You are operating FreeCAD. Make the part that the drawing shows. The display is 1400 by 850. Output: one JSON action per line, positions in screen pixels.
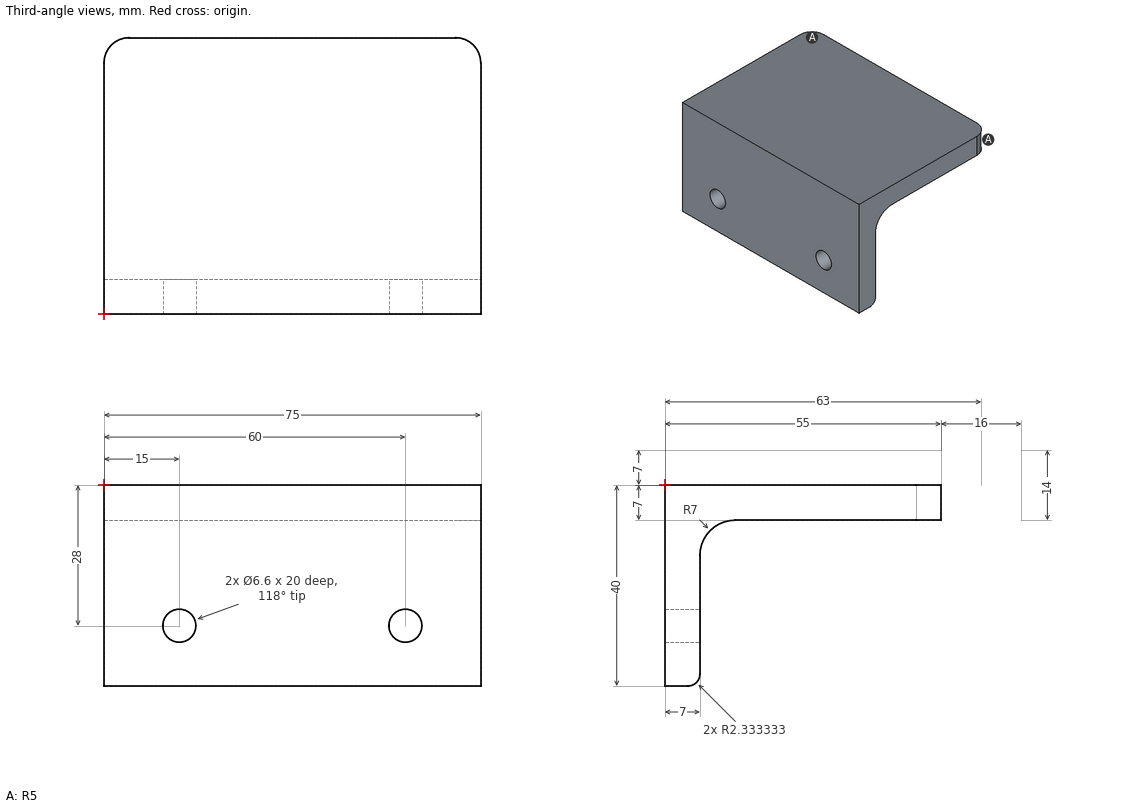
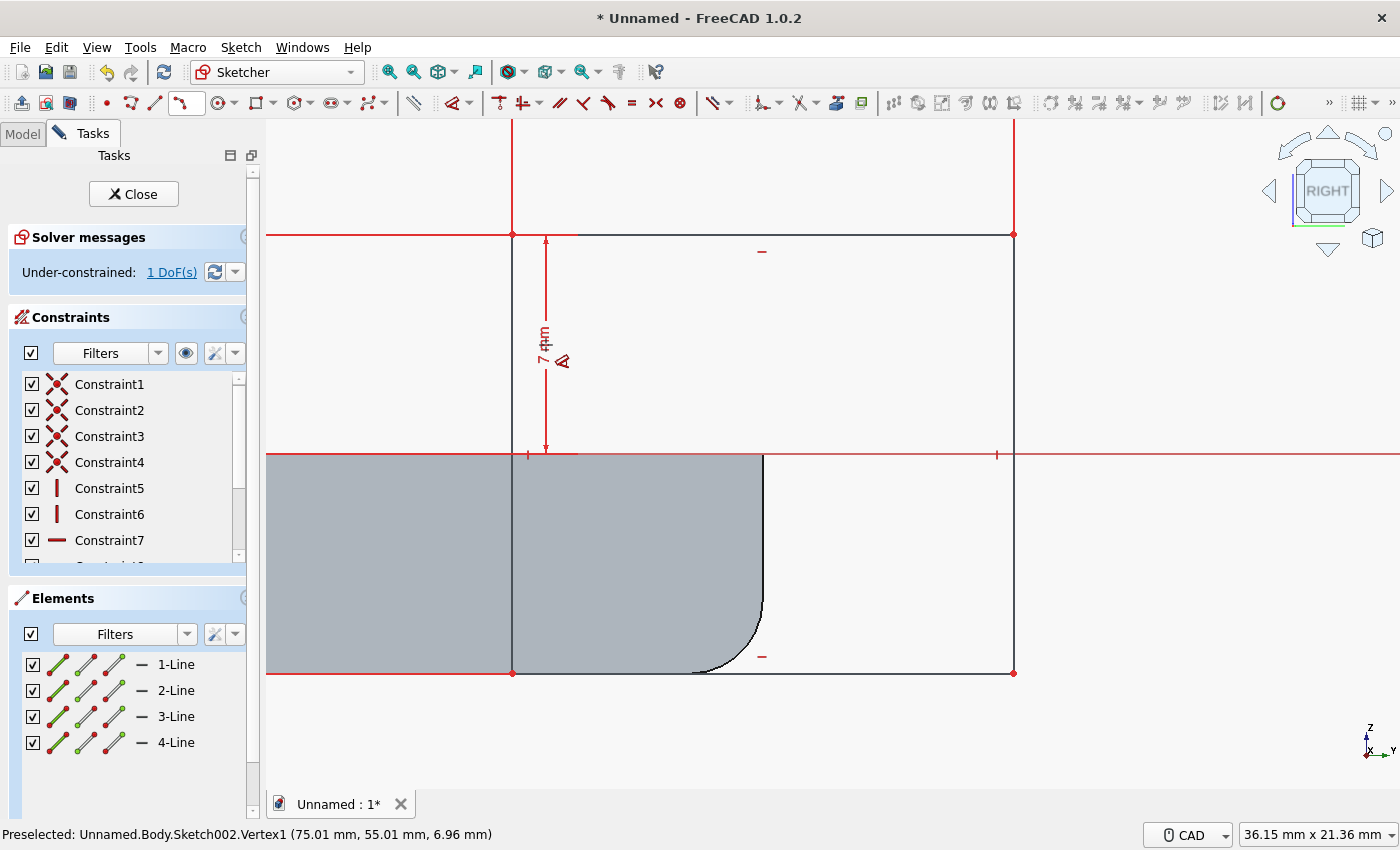
{"action": "left_click", "coordinate": [512, 235]}
{"action": "left_click", "coordinate": [403, 201]}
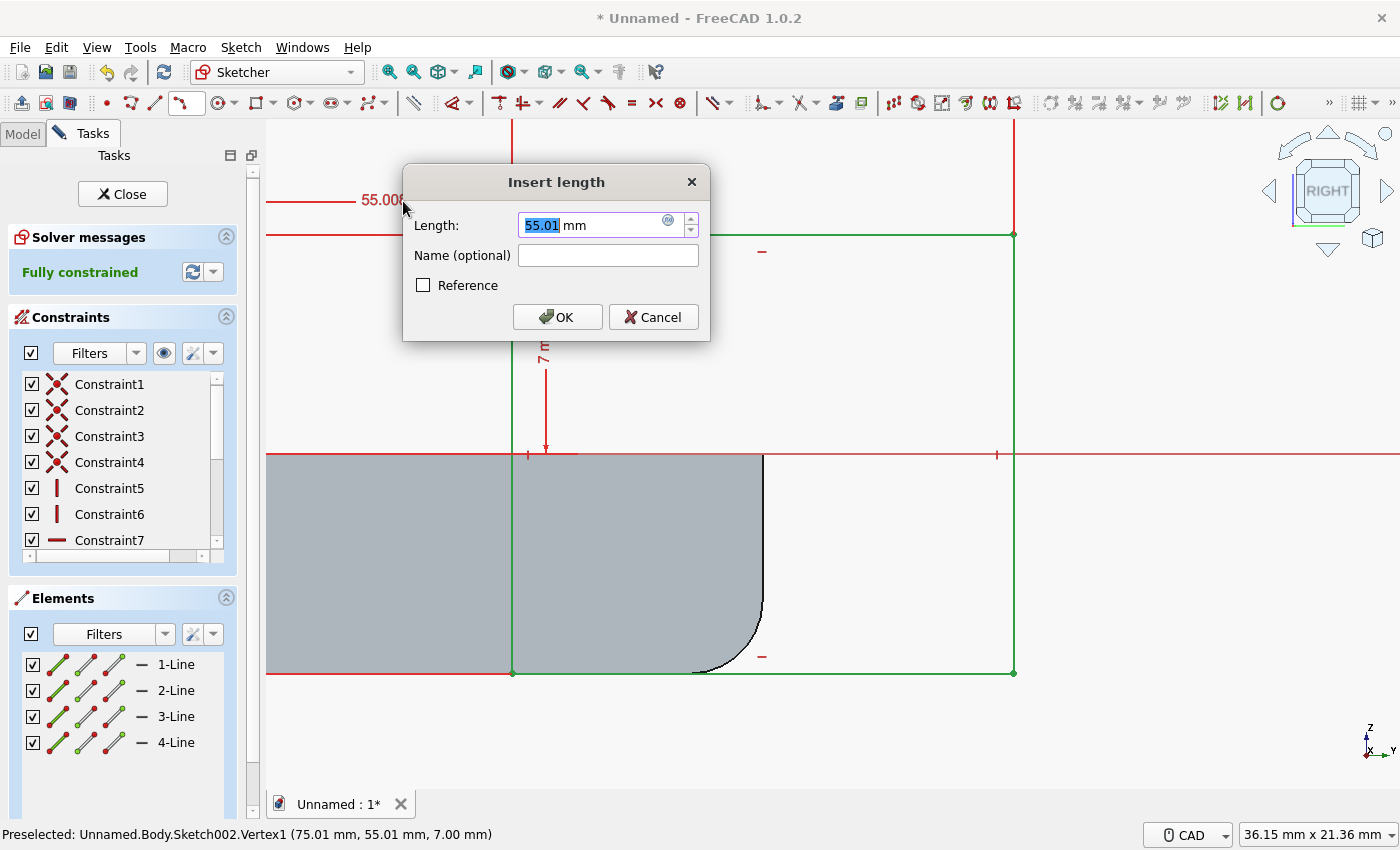
{"action": "type", "text": "55"}
{"action": "key", "text": "Return"}
{"action": "key", "text": "Escape"}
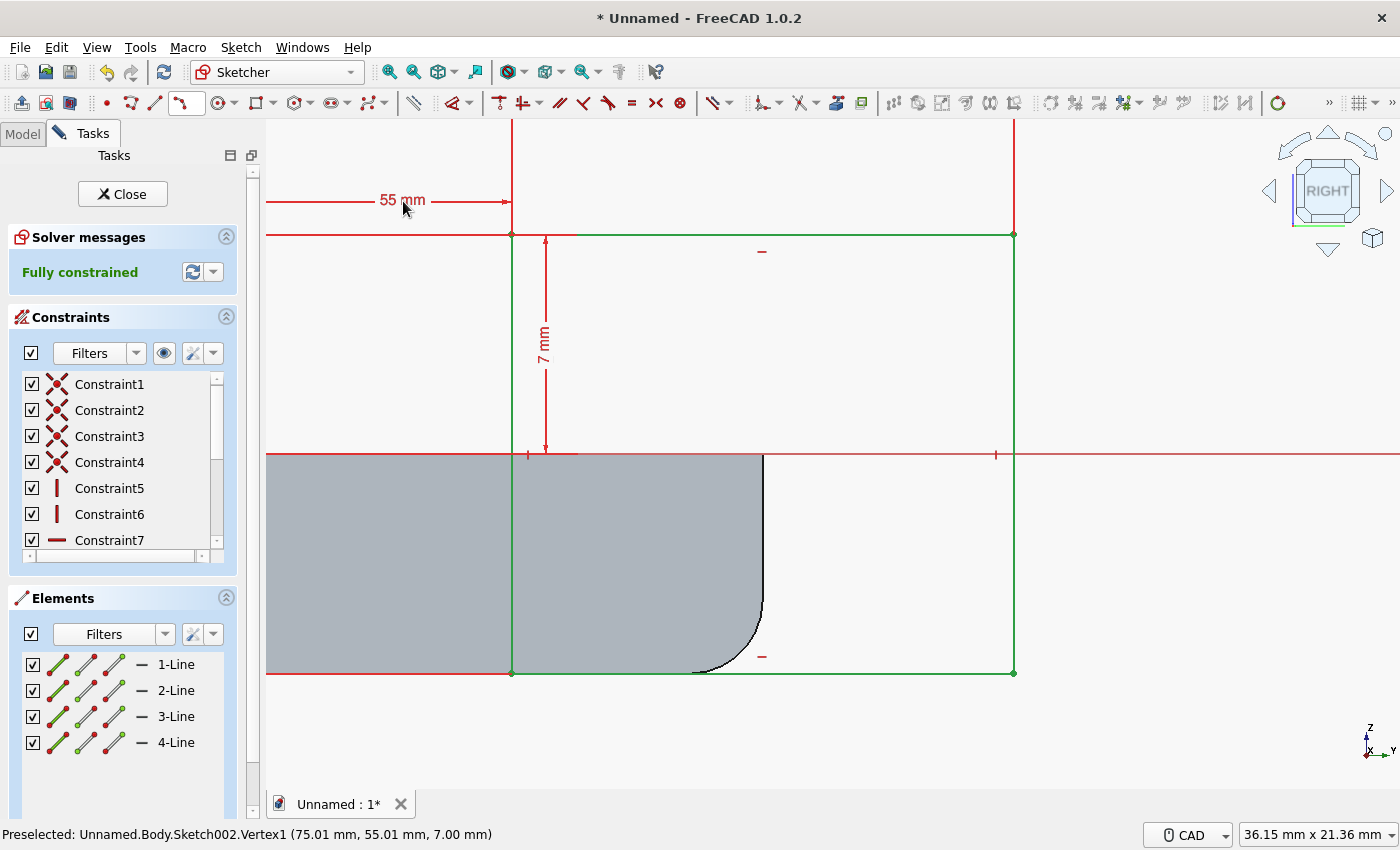
{"action": "left_click", "coordinate": [123, 194]}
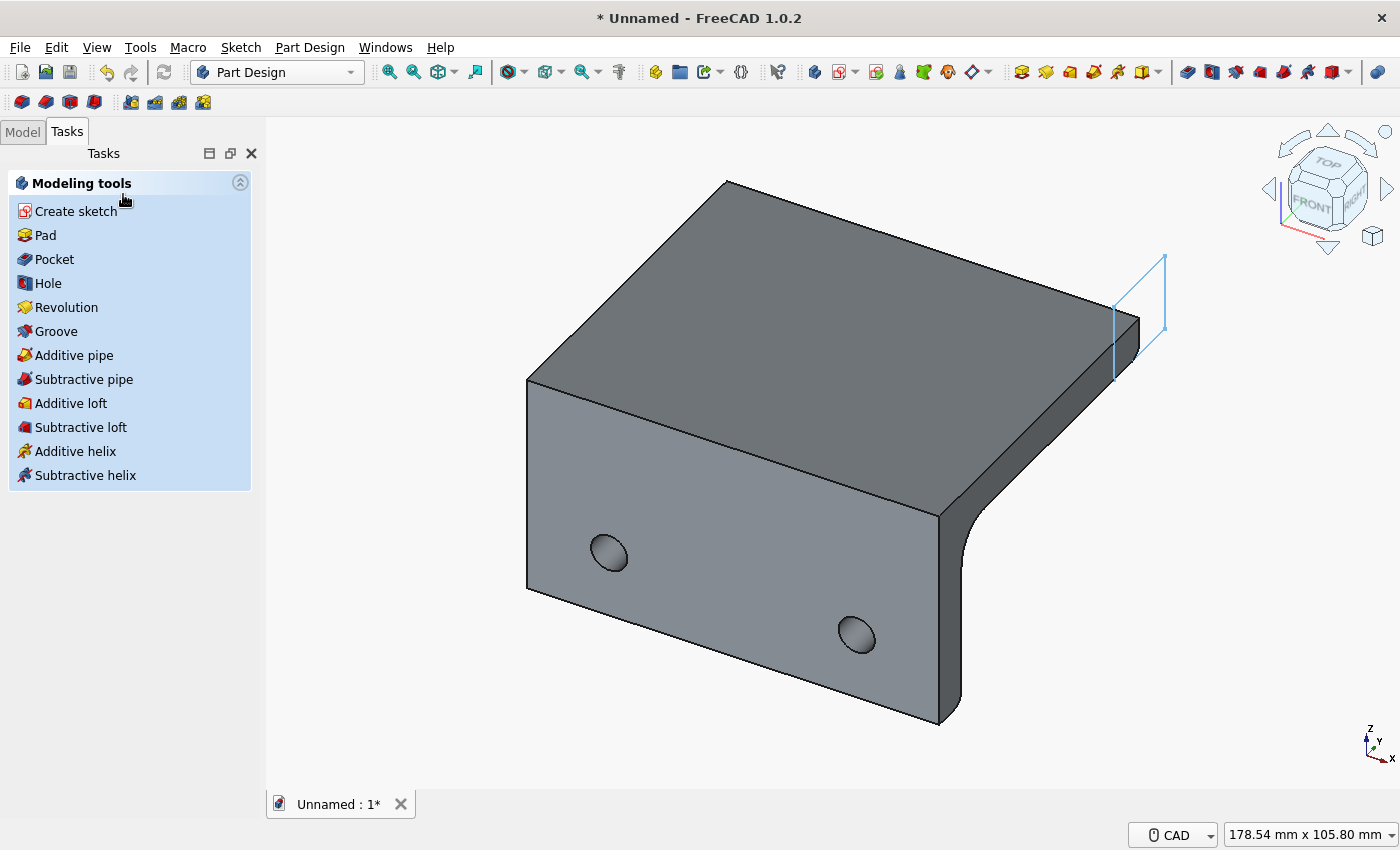
{"action": "left_click", "coordinate": [1188, 72]}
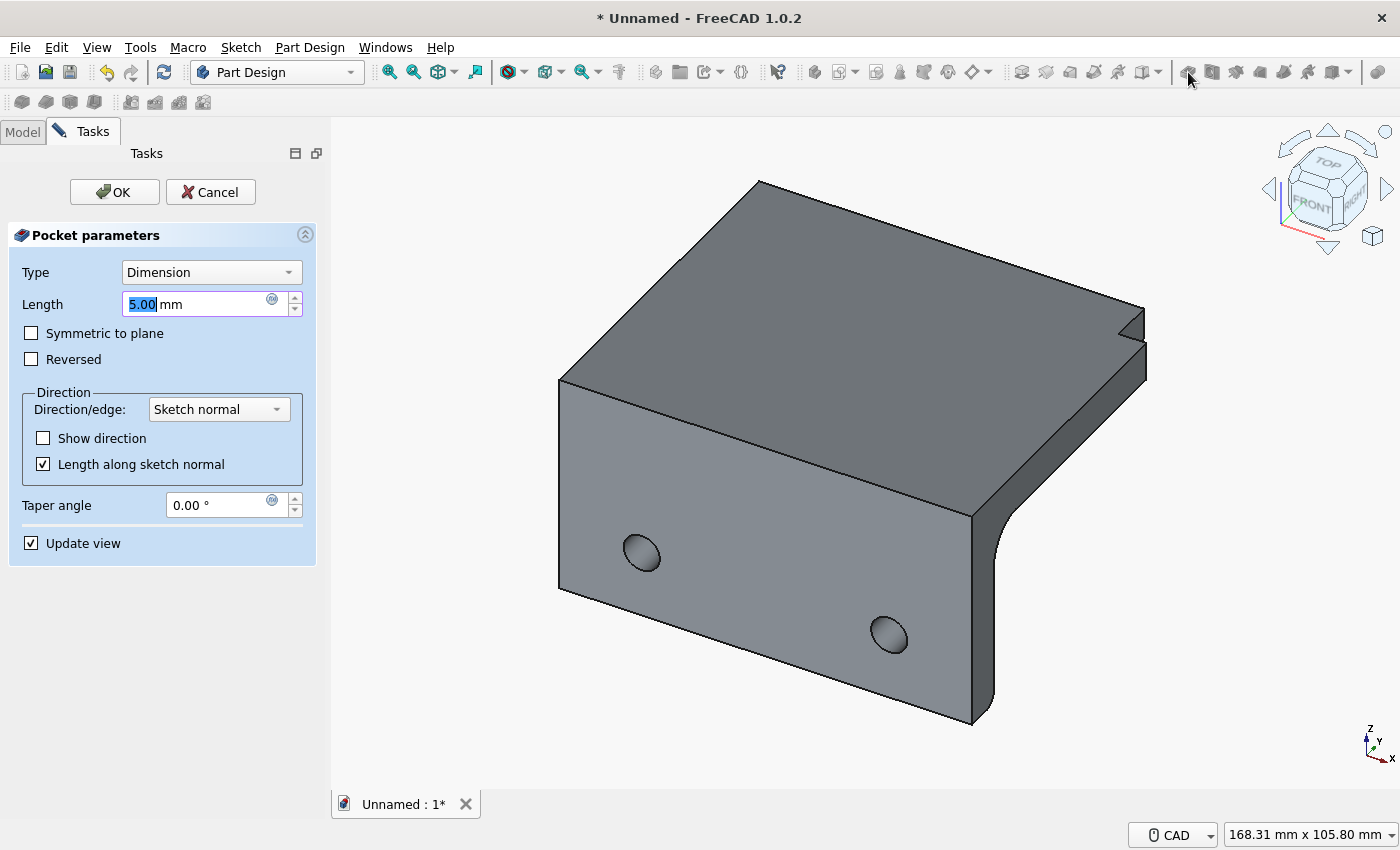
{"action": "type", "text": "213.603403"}
{"action": "key", "text": "Tab"}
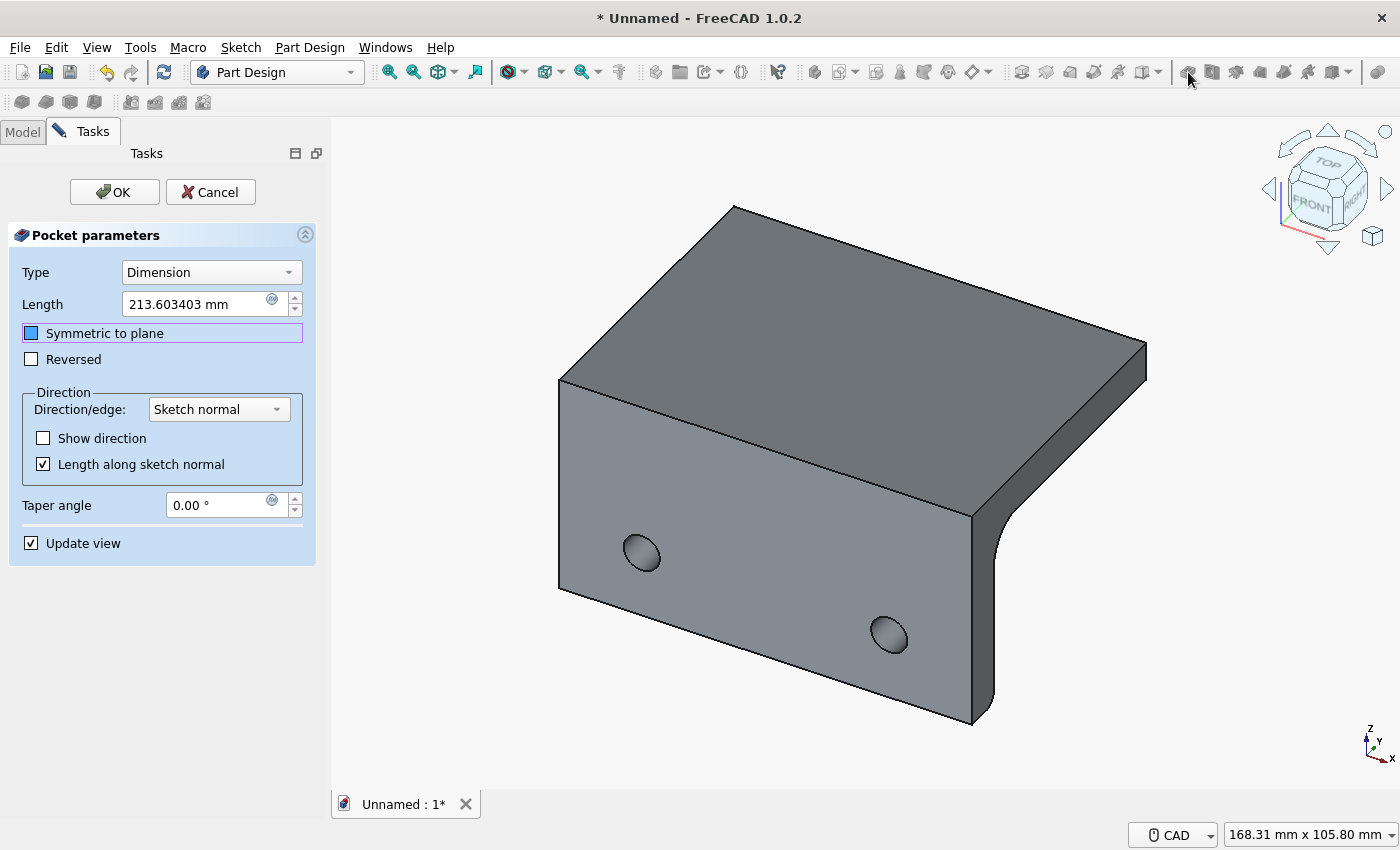
{"action": "left_click", "coordinate": [30, 333]}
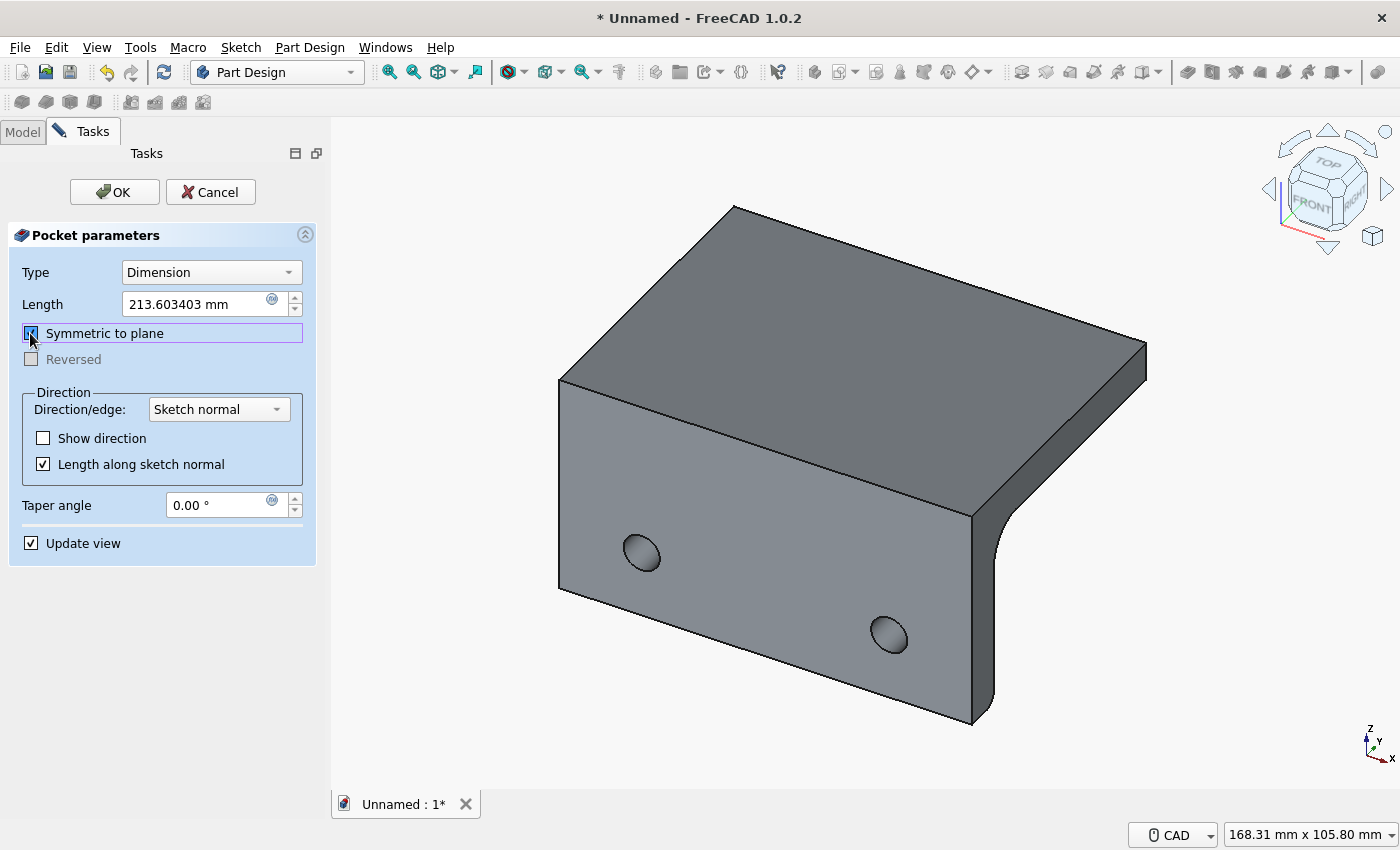
{"action": "left_click", "coordinate": [115, 192]}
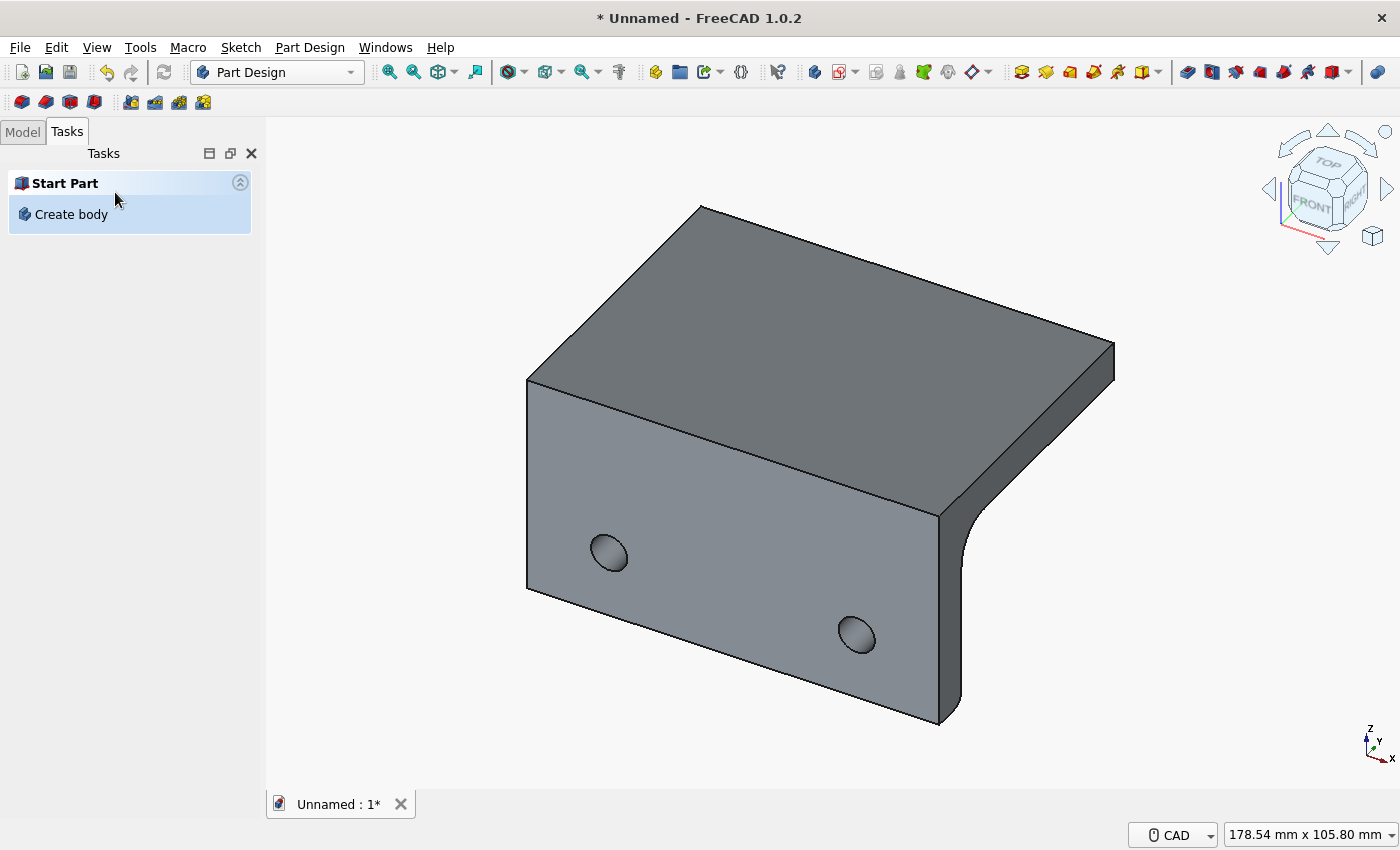
{"action": "key", "text": "0"}